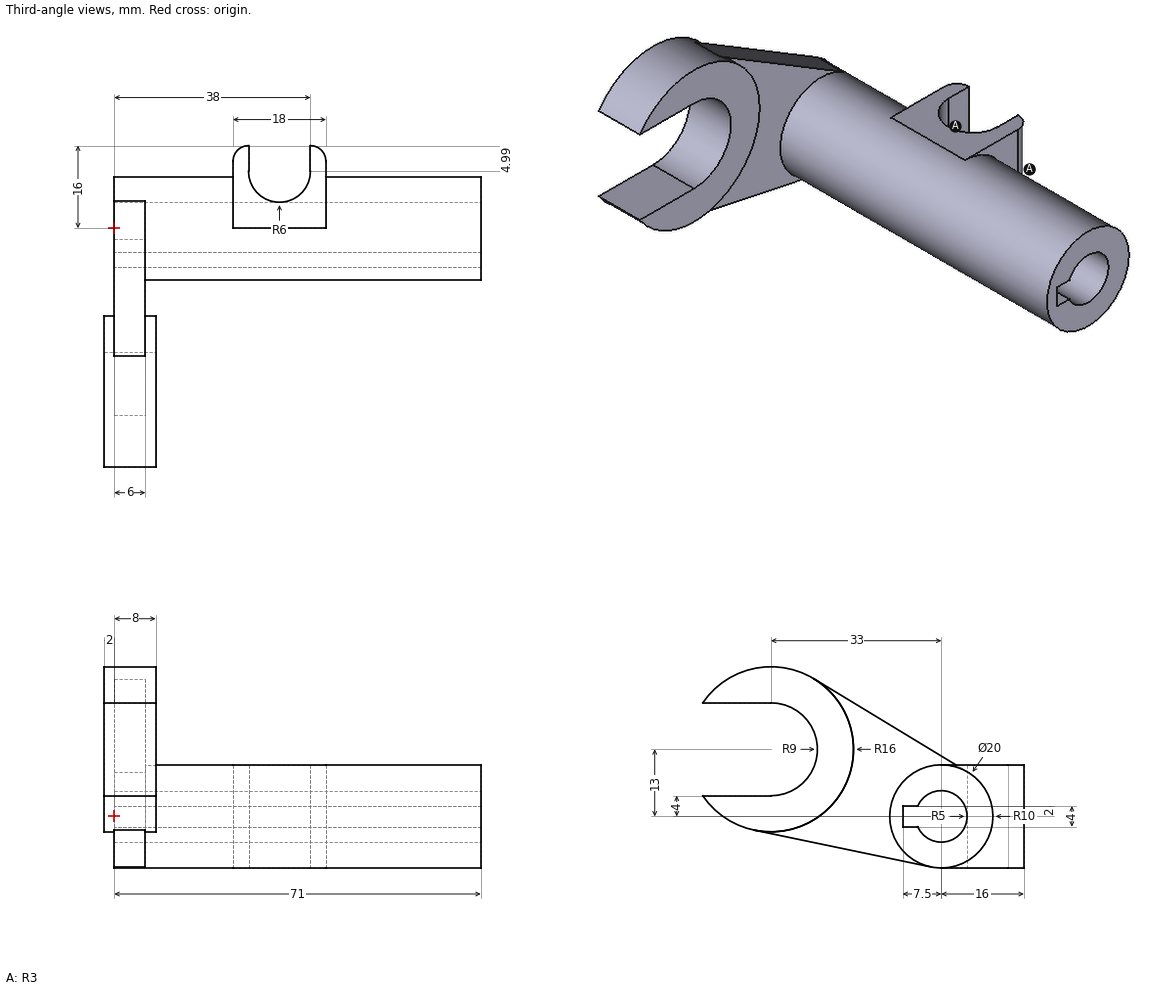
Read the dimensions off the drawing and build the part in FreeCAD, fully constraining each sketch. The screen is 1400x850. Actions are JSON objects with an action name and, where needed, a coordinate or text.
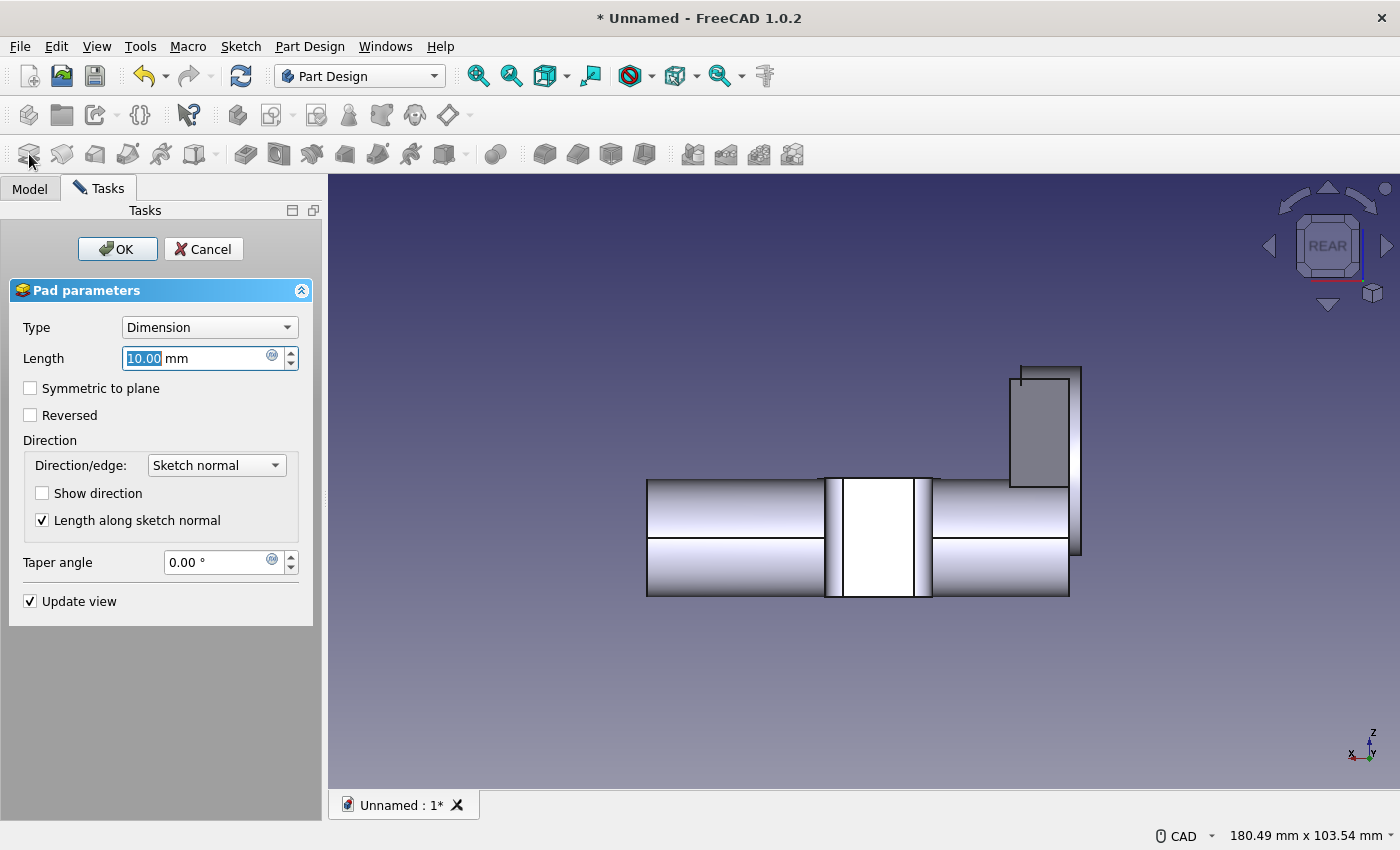
{"action": "type", "text": "6"}
{"action": "key", "text": "Tab"}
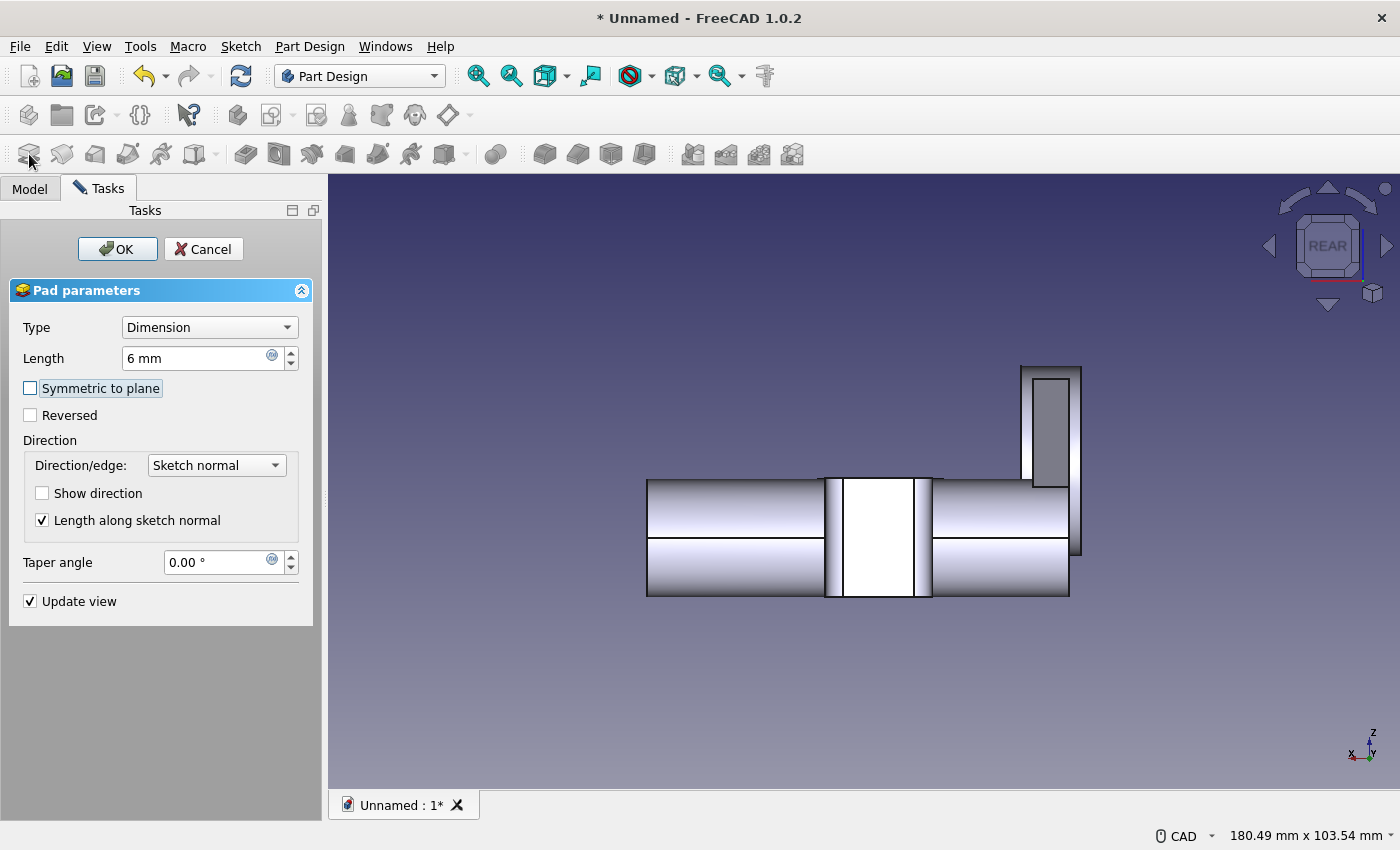
{"action": "left_click", "coordinate": [118, 249]}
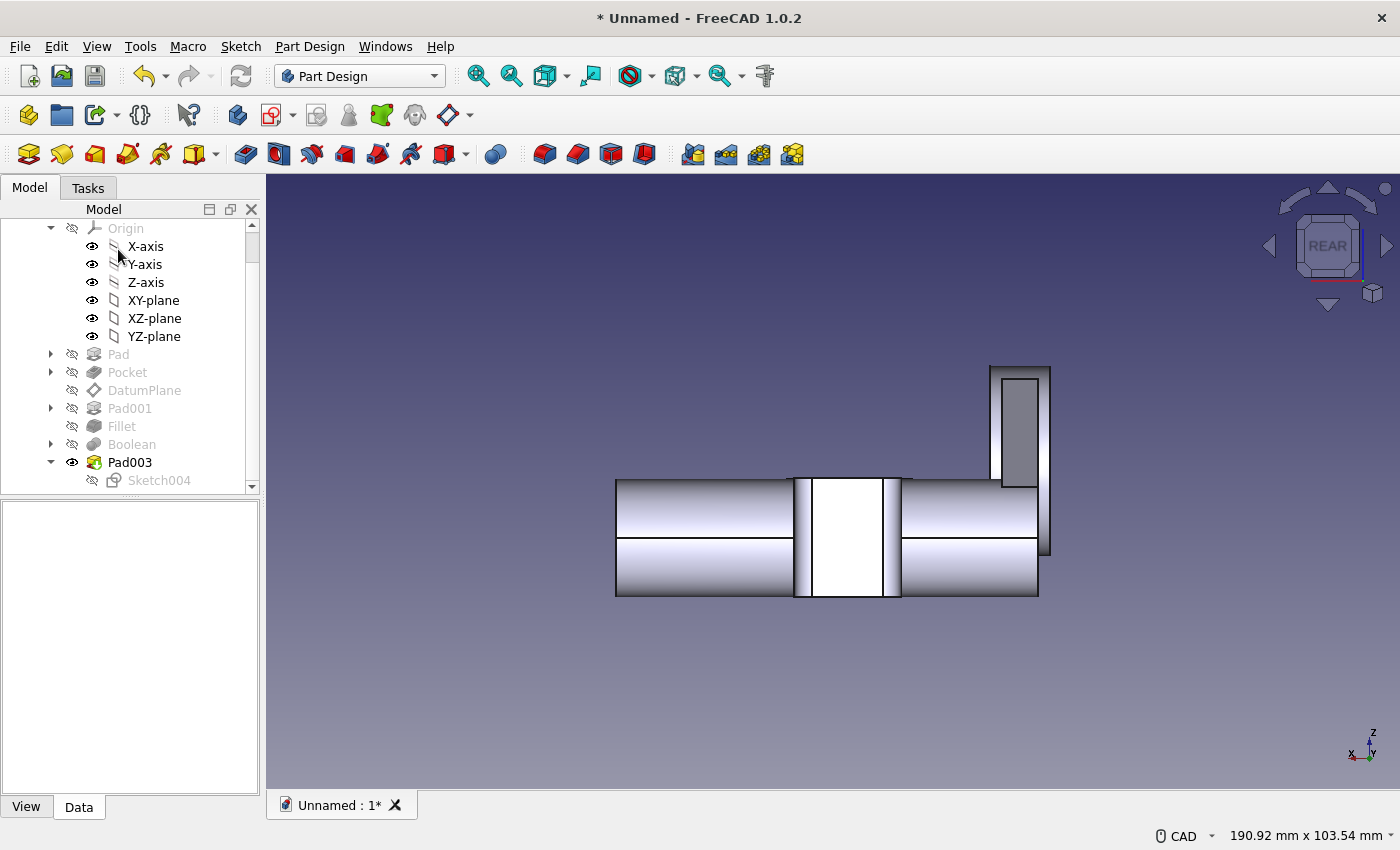
{"action": "left_click", "coordinate": [479, 76]}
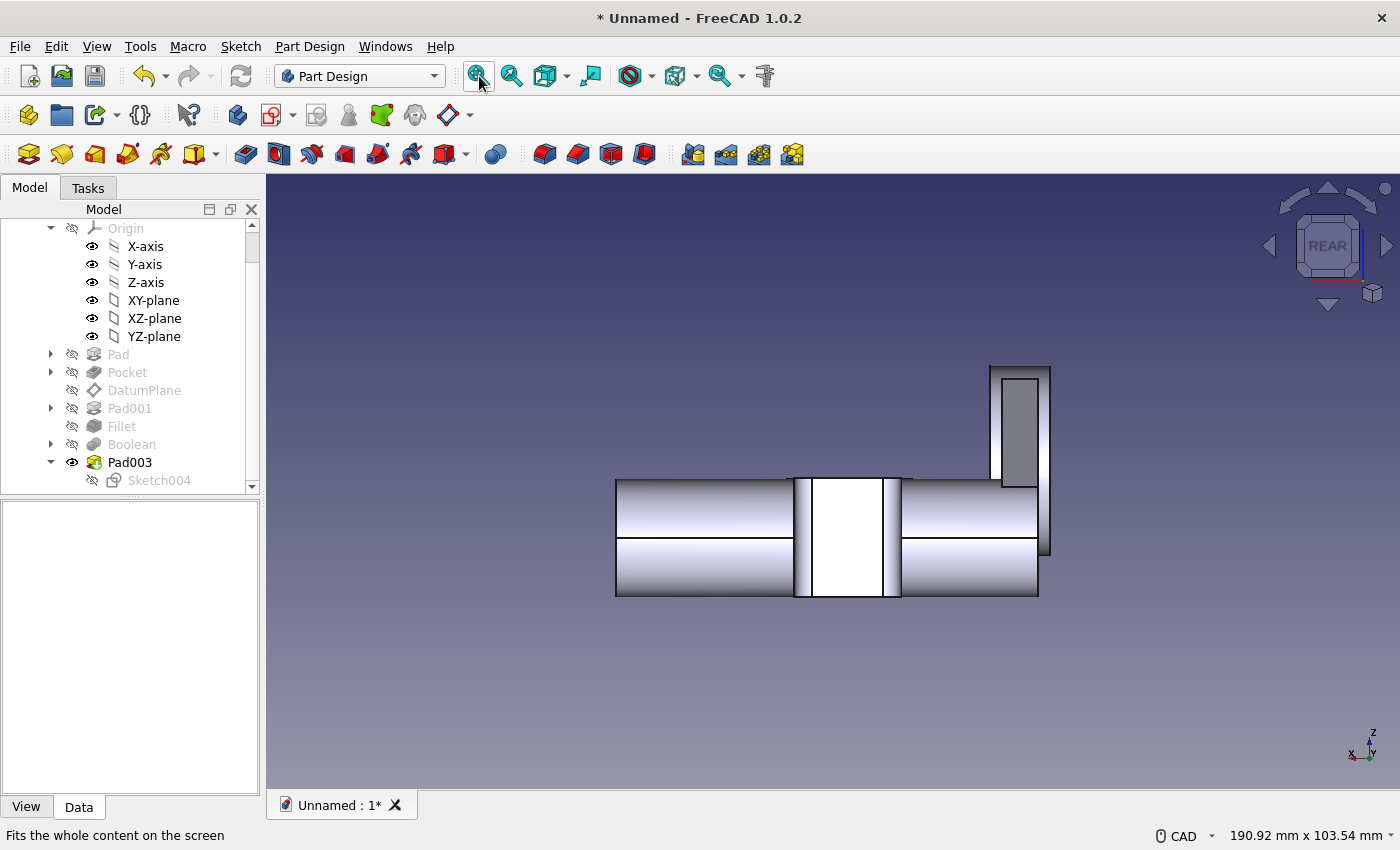
{"action": "left_click", "coordinate": [270, 116]}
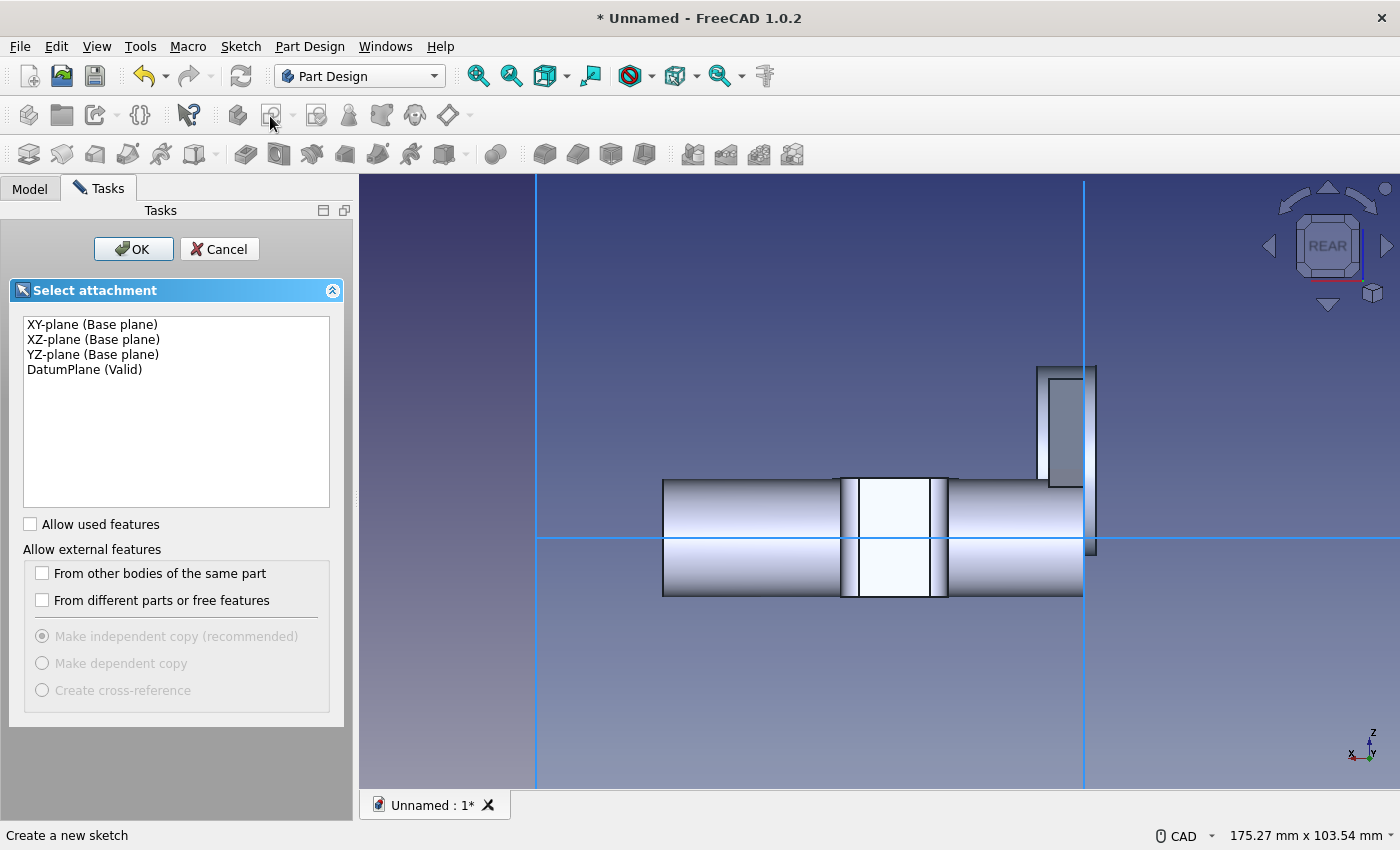
{"action": "left_click", "coordinate": [84, 324]}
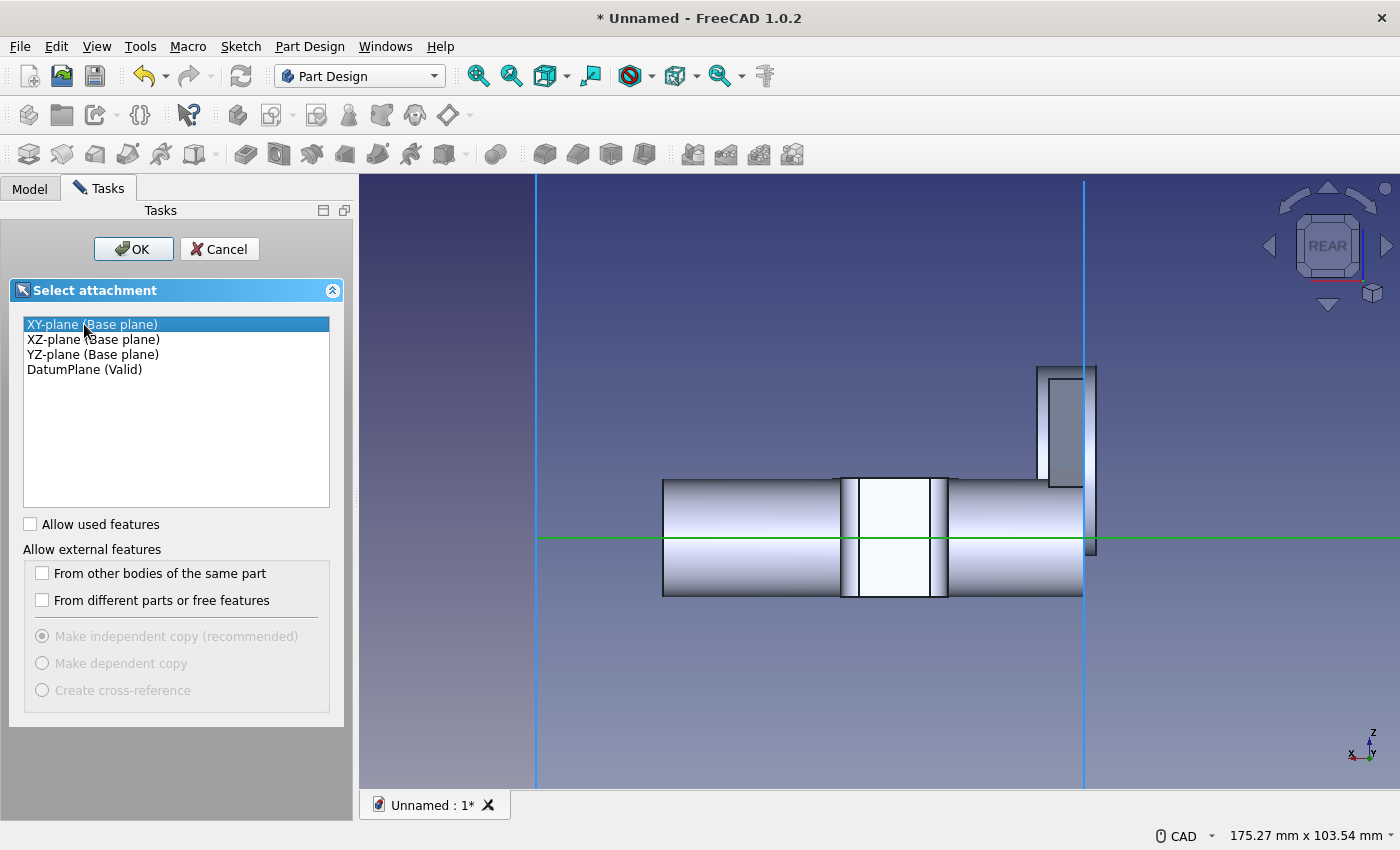
{"action": "left_click", "coordinate": [134, 249]}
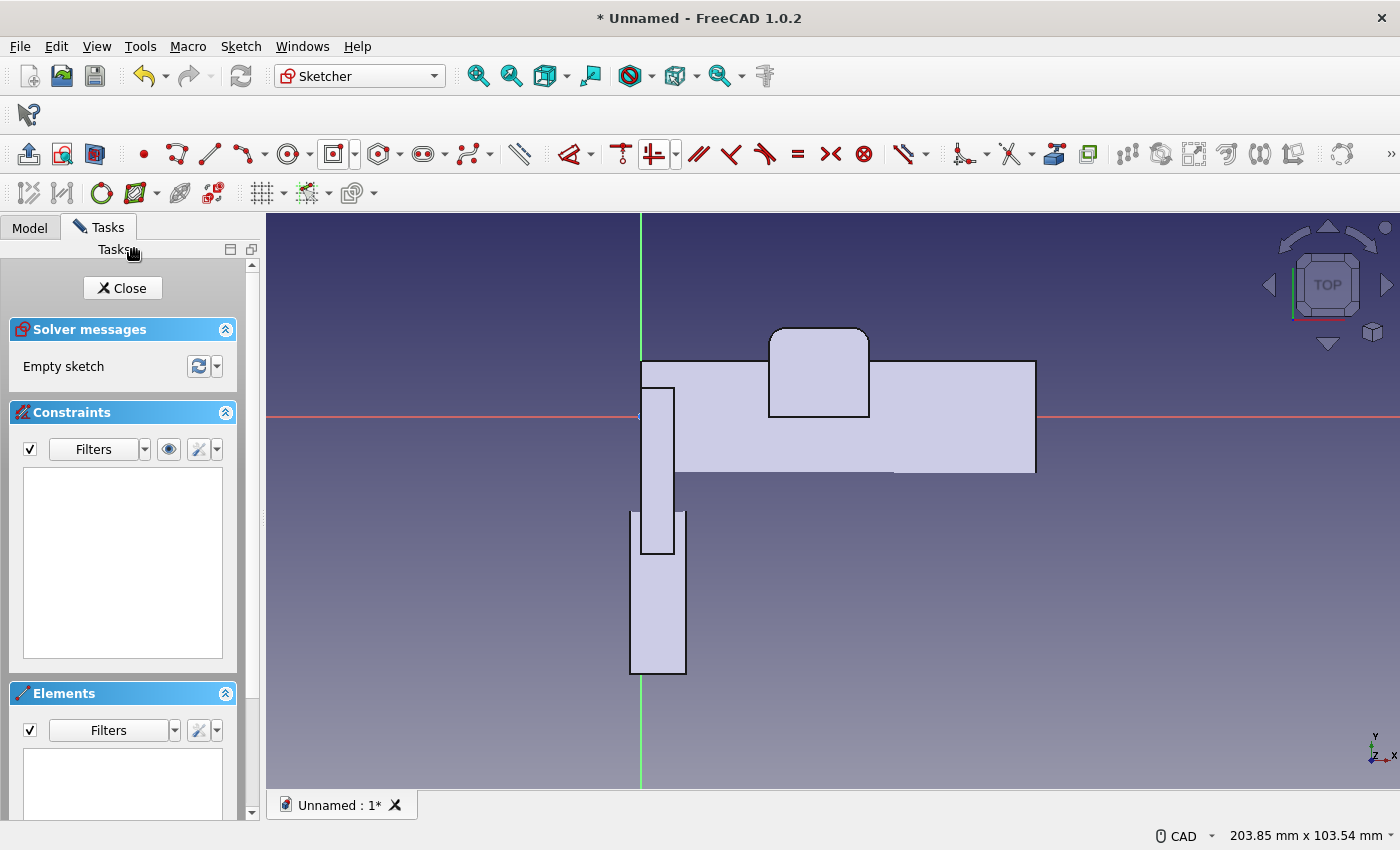
{"action": "left_click", "coordinate": [95, 154]}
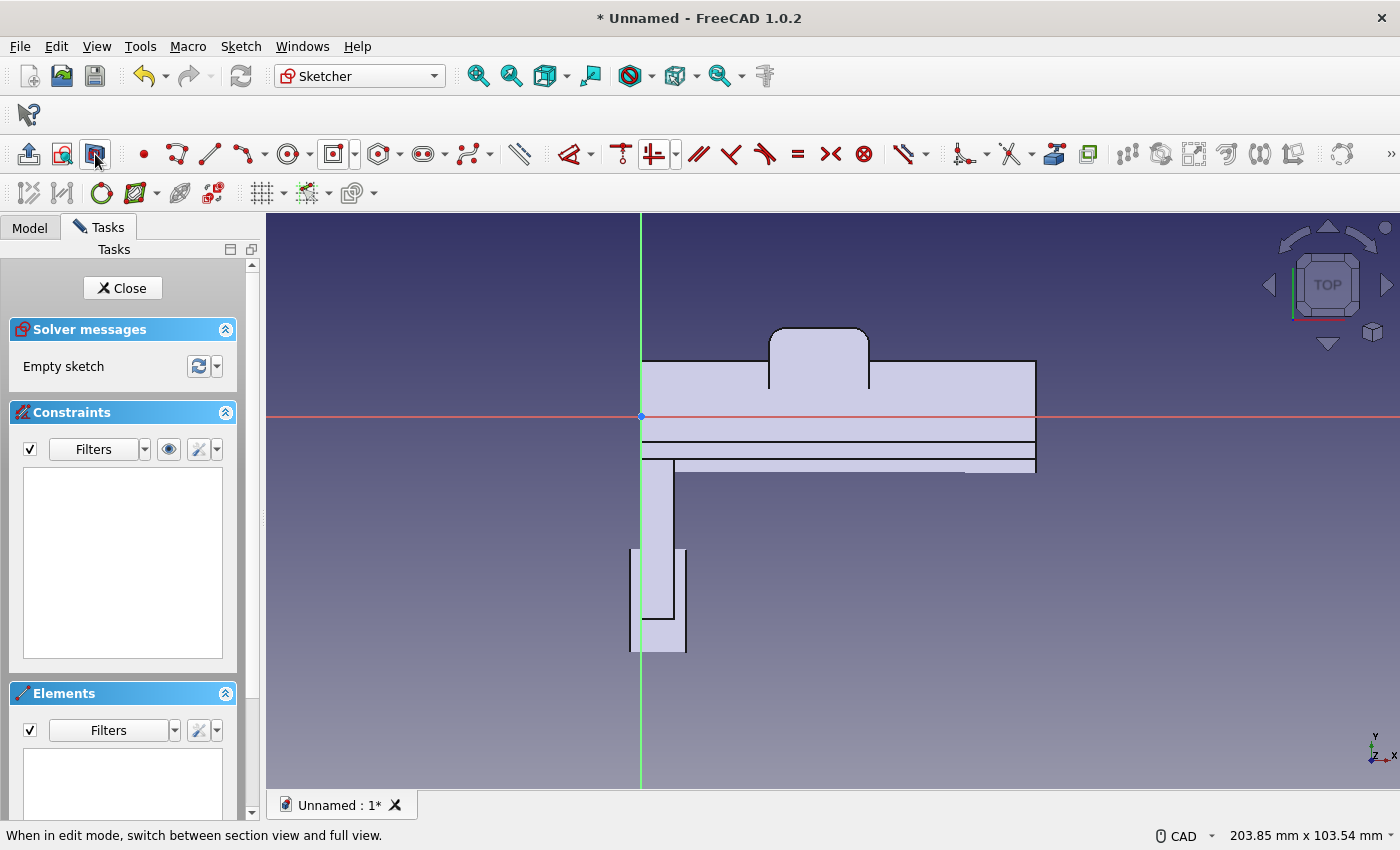
{"action": "scroll", "coordinate": [830, 330], "scroll_direction": "up", "scroll_amount": 9}